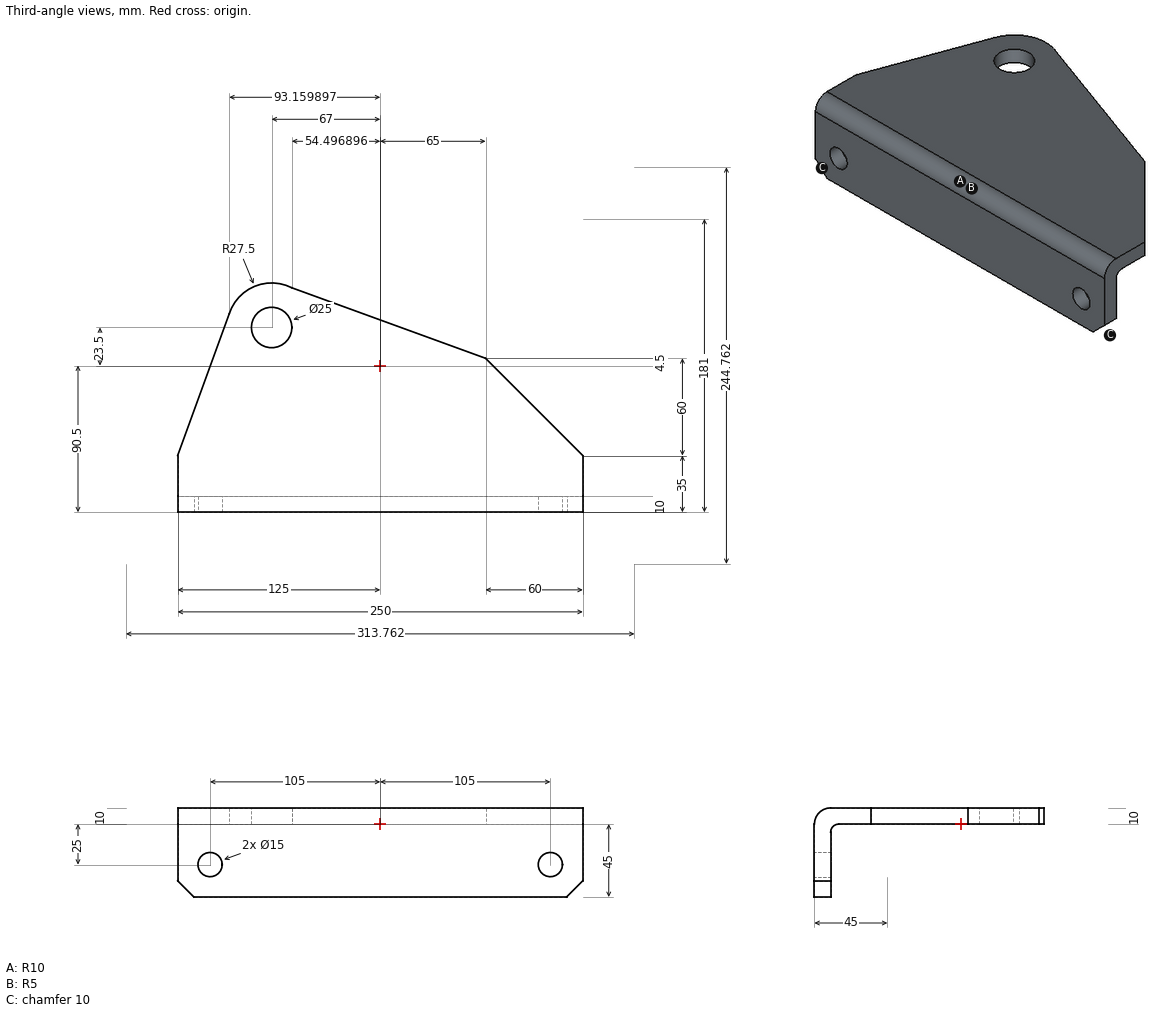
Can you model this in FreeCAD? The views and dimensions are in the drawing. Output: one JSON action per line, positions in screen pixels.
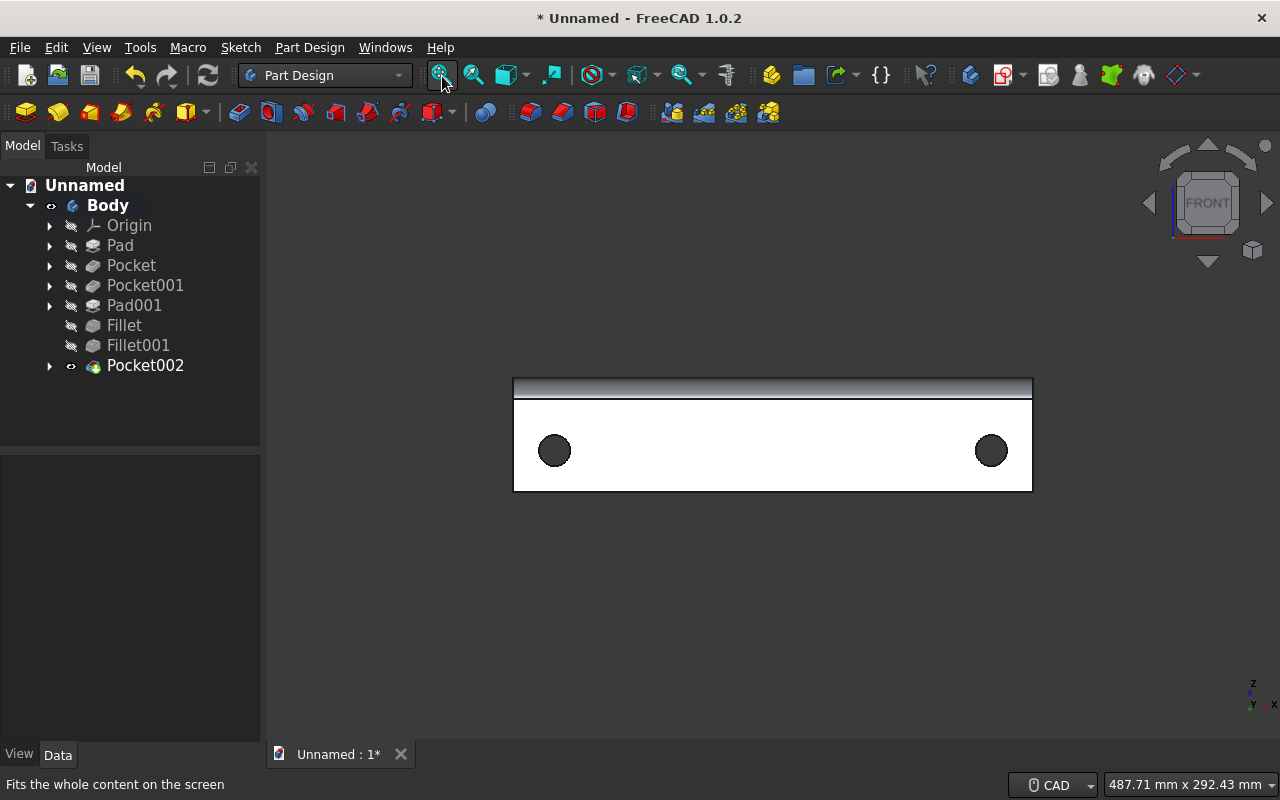
{"action": "key", "text": "3"}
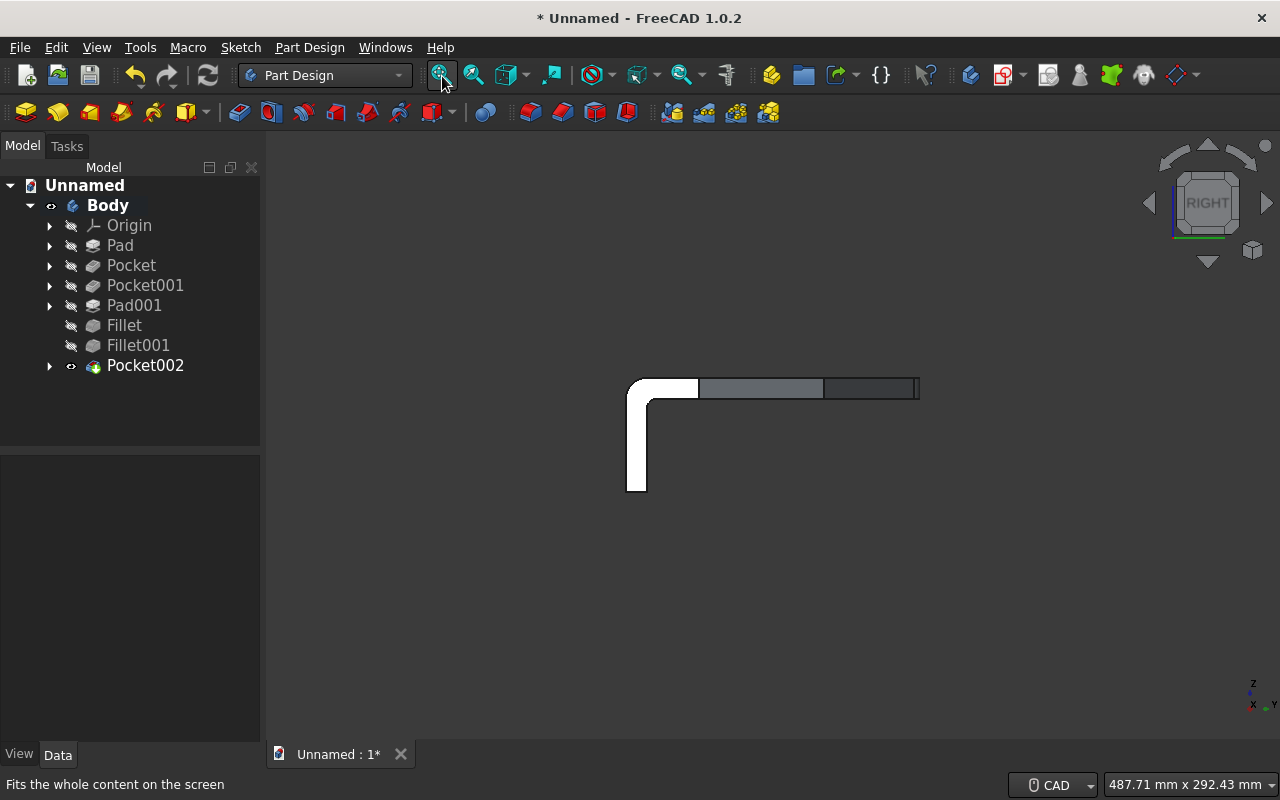
{"action": "key", "text": "v f"}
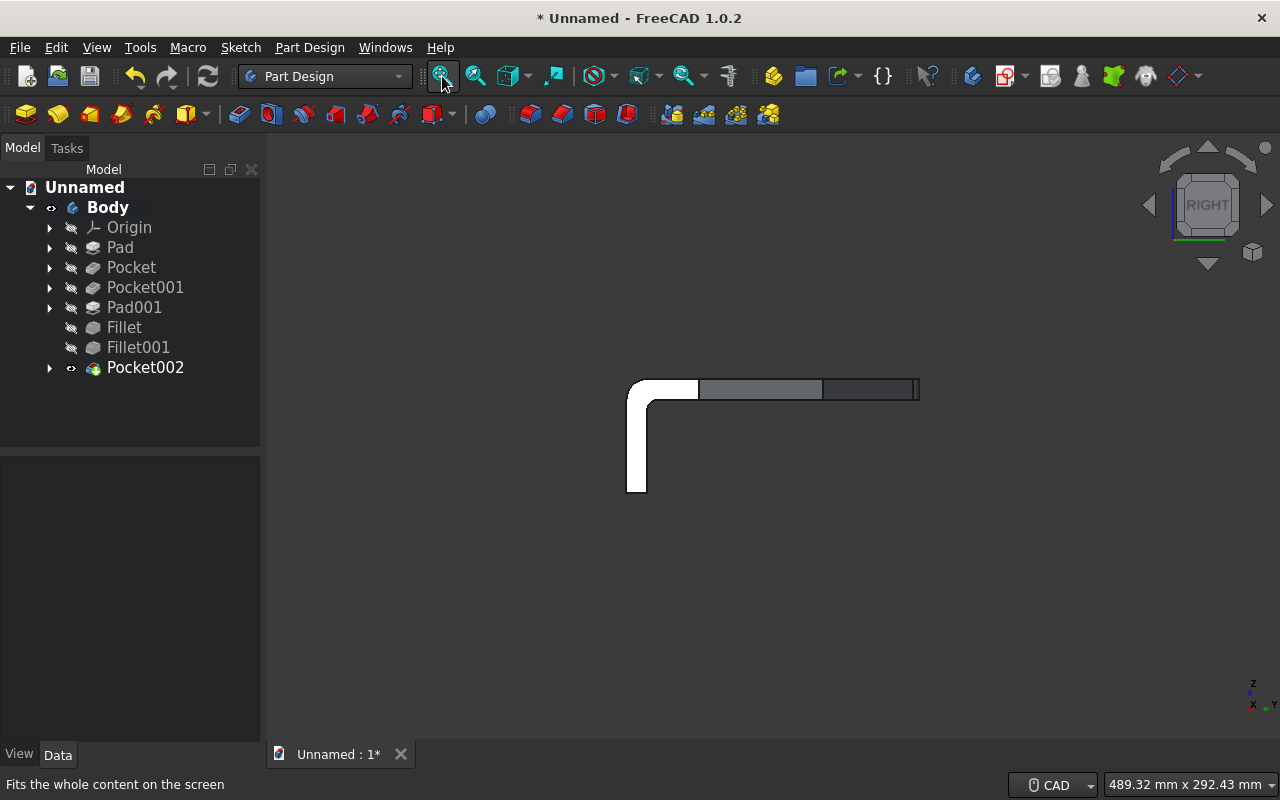
{"action": "left_click", "coordinate": [637, 492]}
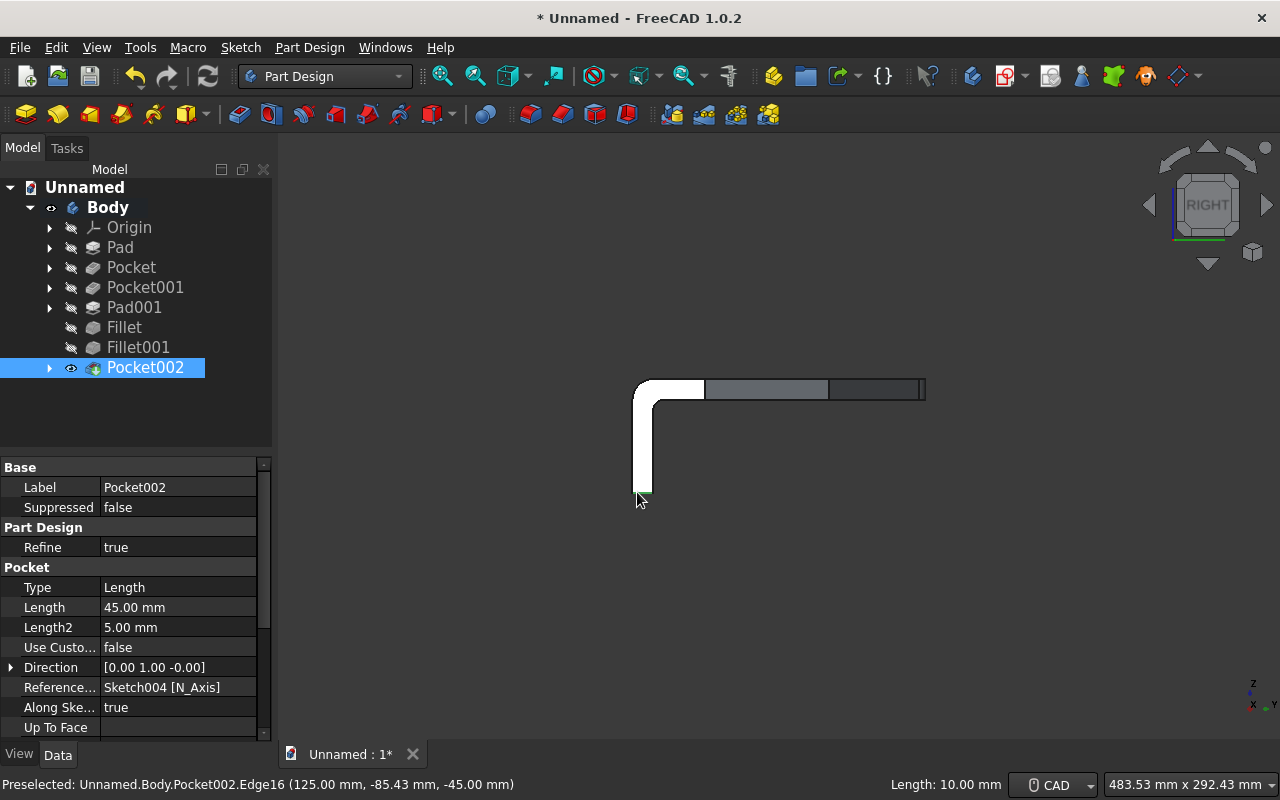
{"action": "scroll", "coordinate": [643, 492], "scroll_direction": "up", "scroll_amount": 4}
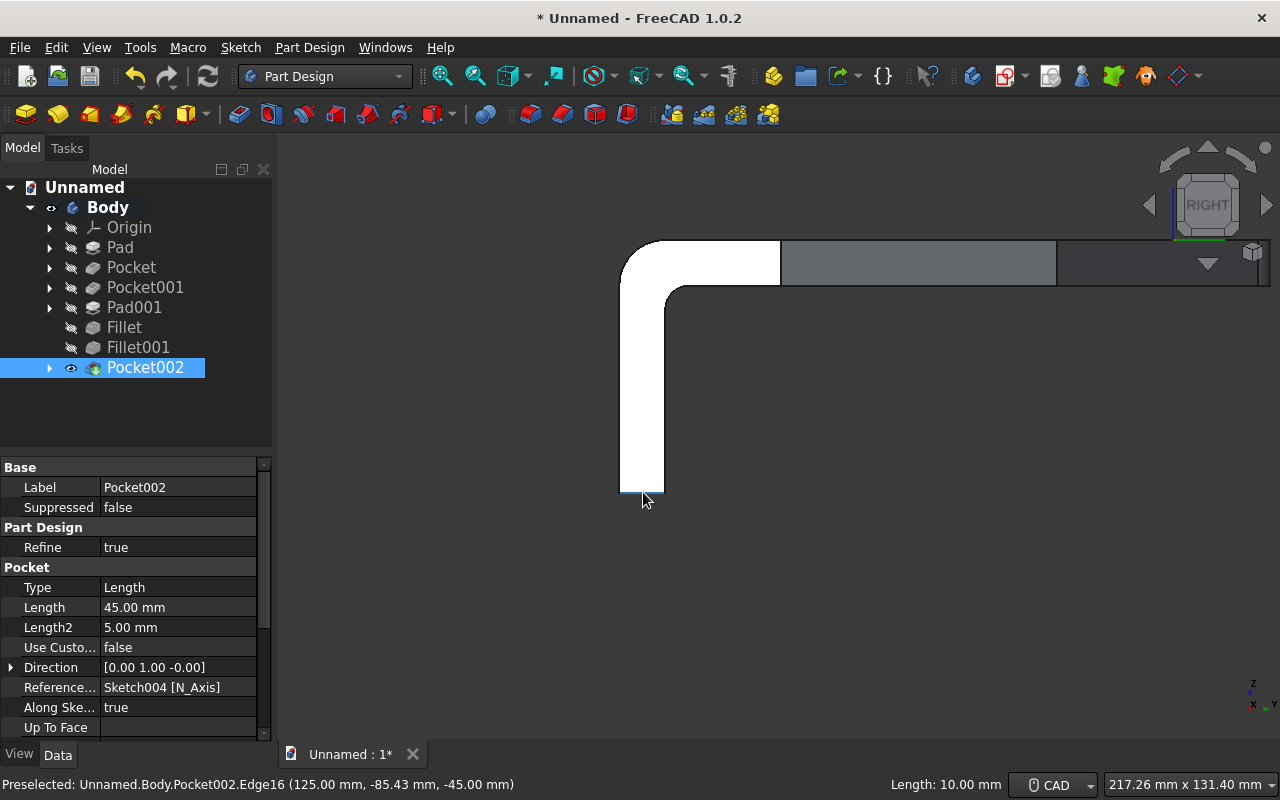
{"action": "key", "text": "v f"}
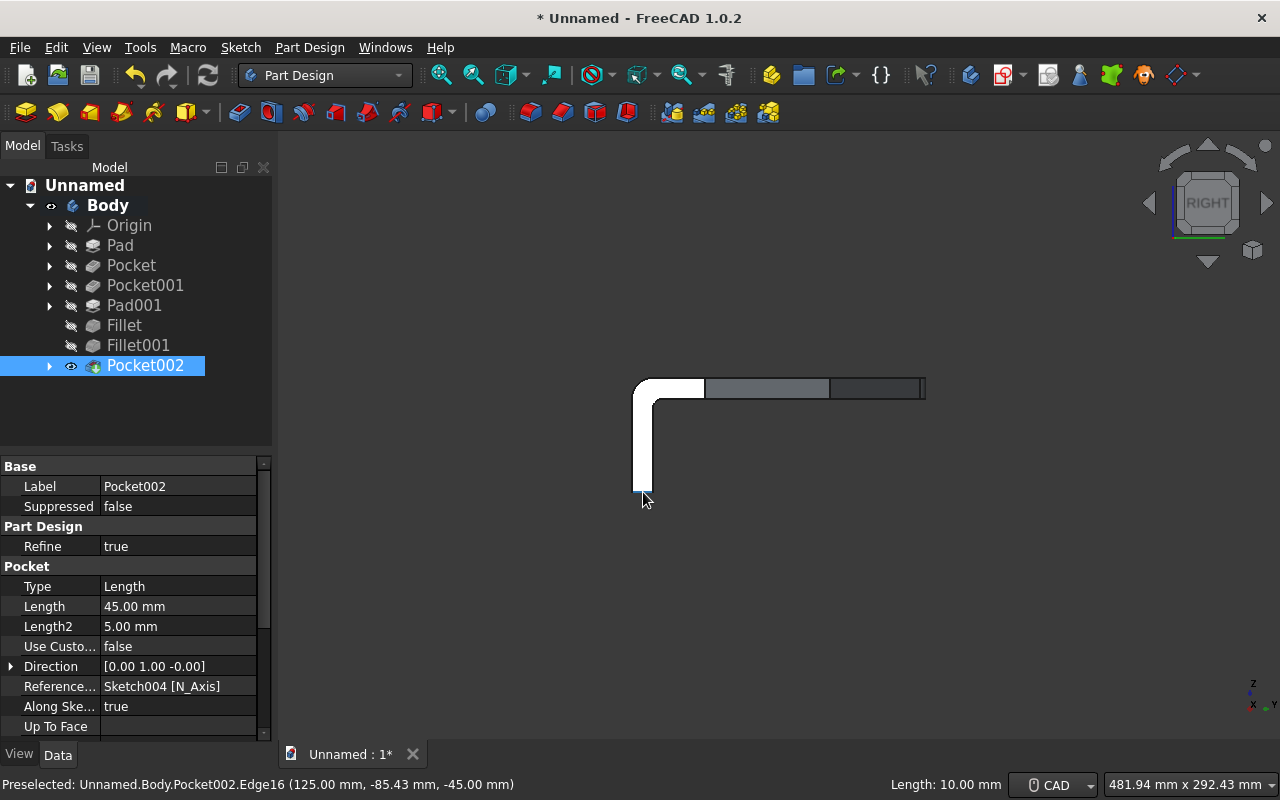
{"action": "key", "text": "5"}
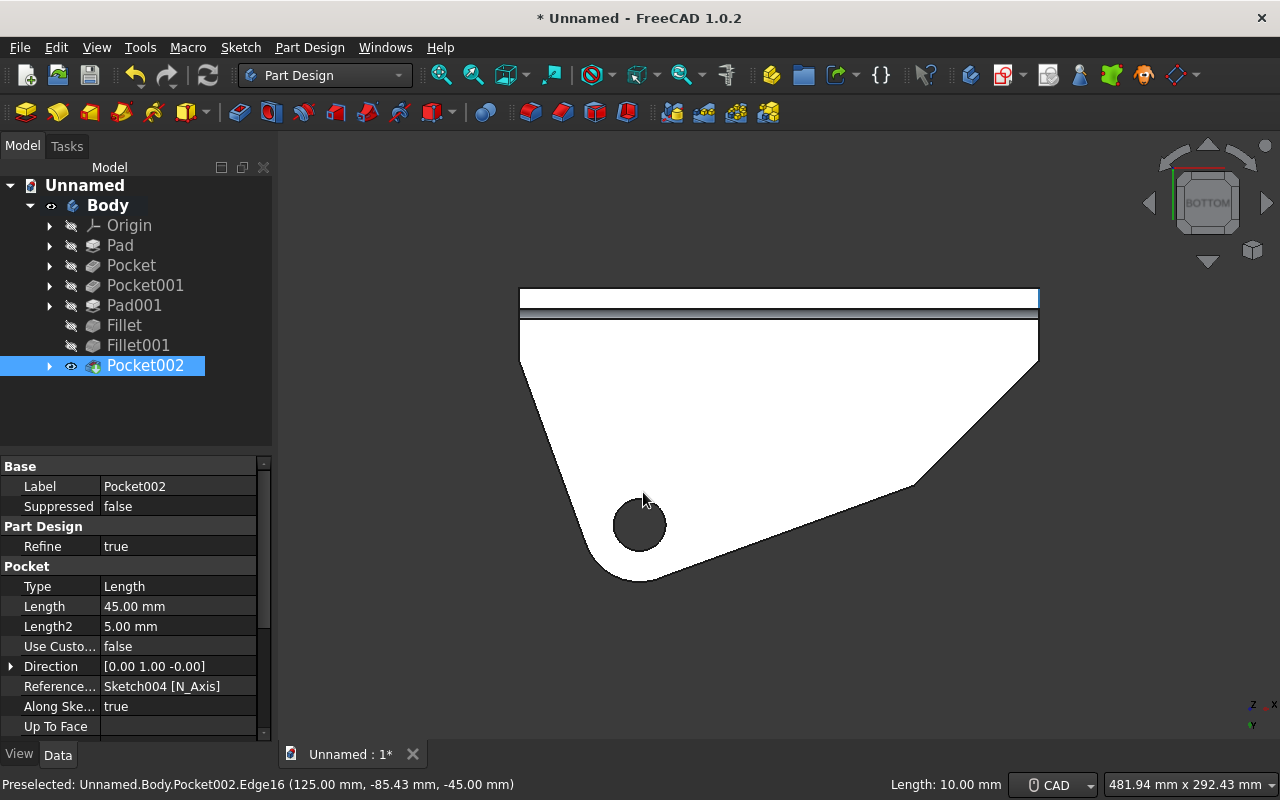
{"action": "left_click", "coordinate": [519, 297], "text": "ctrl"}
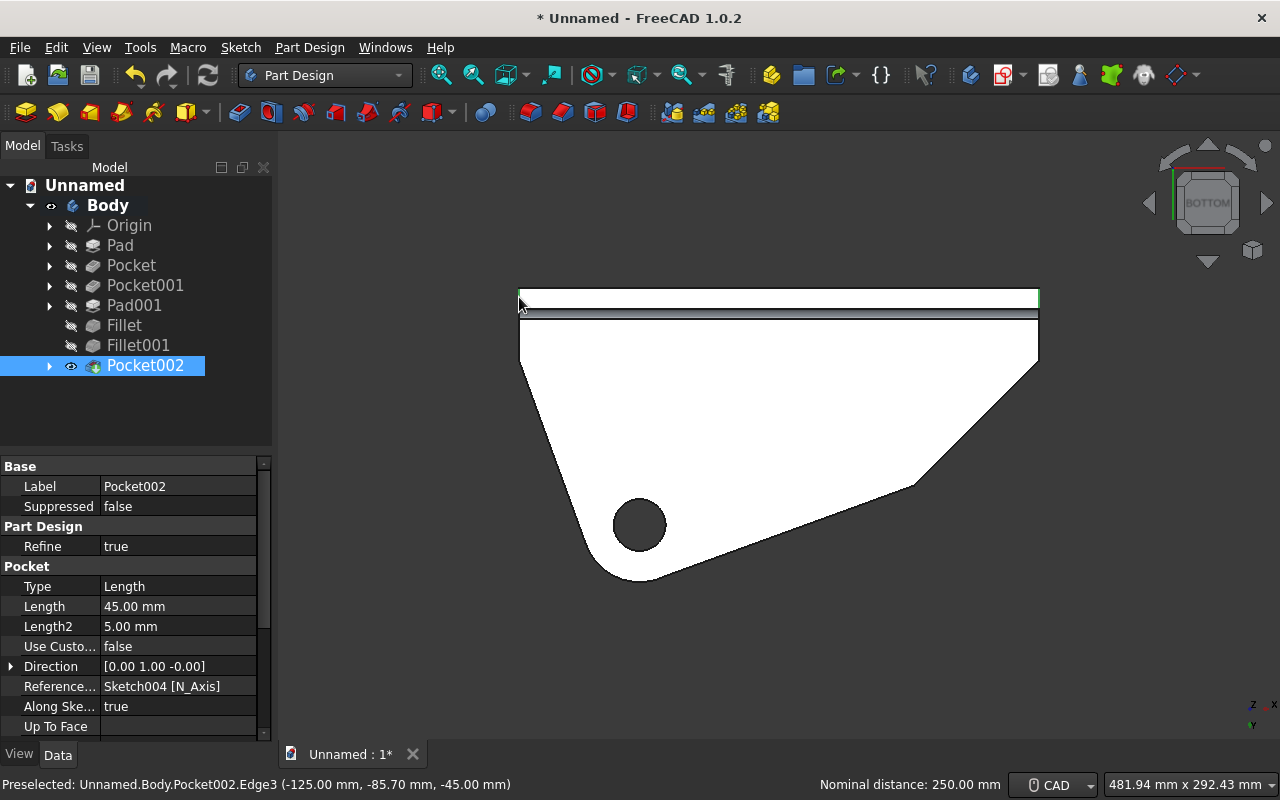
{"action": "left_click", "coordinate": [564, 112]}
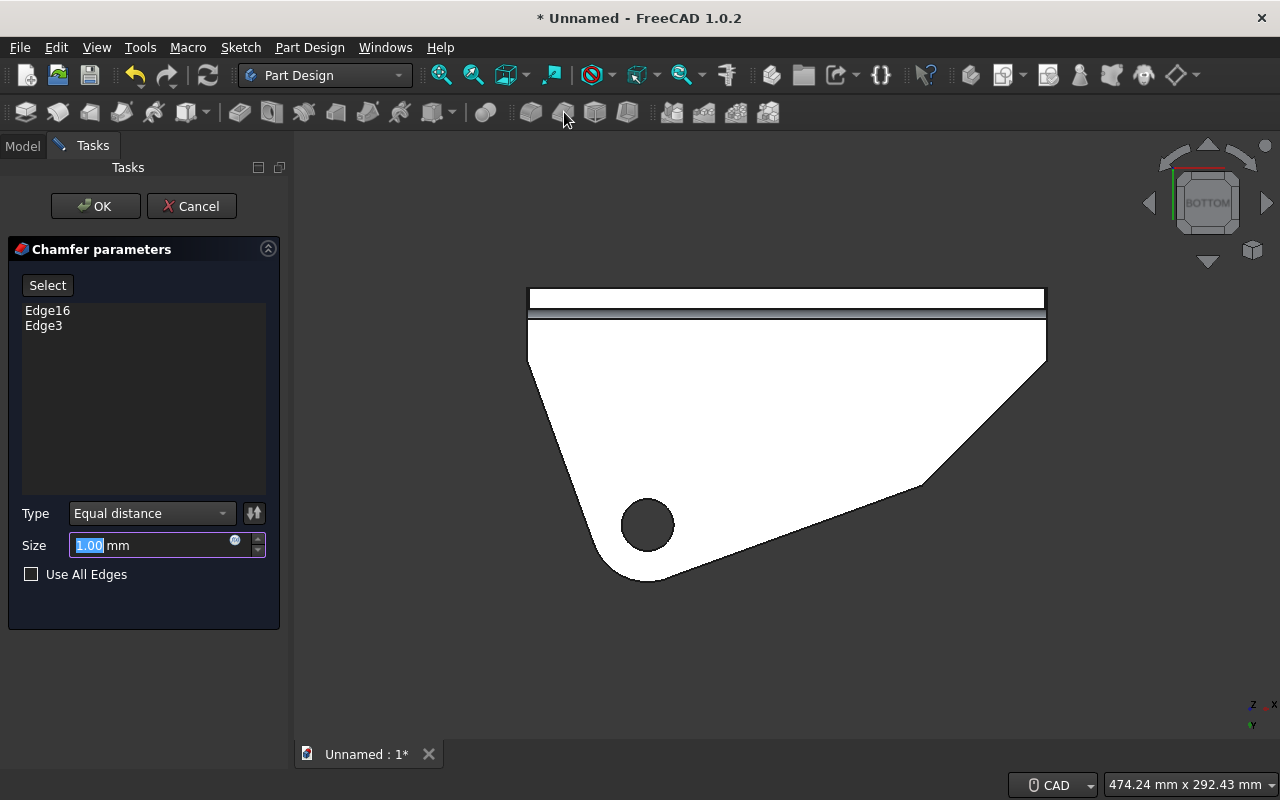
{"action": "type", "text": "10"}
{"action": "key", "text": "Tab"}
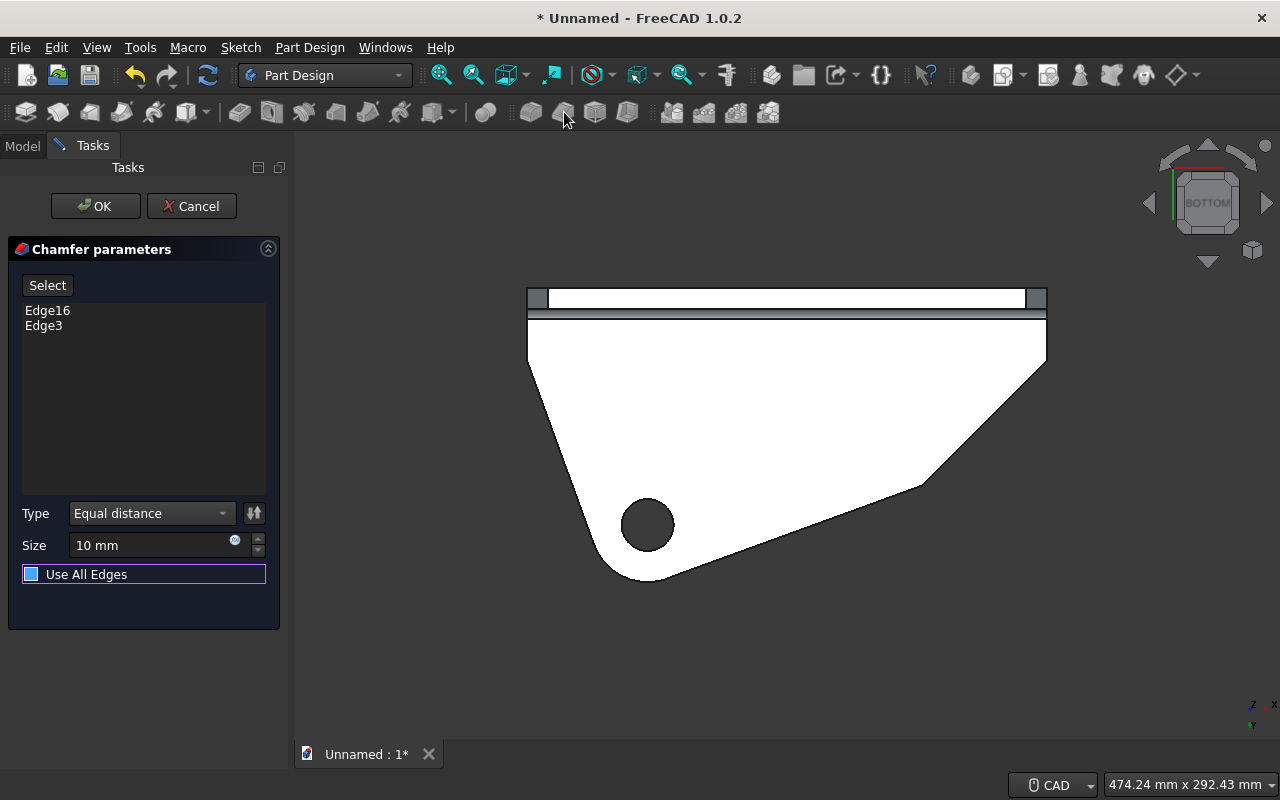
{"action": "left_click", "coordinate": [96, 206]}